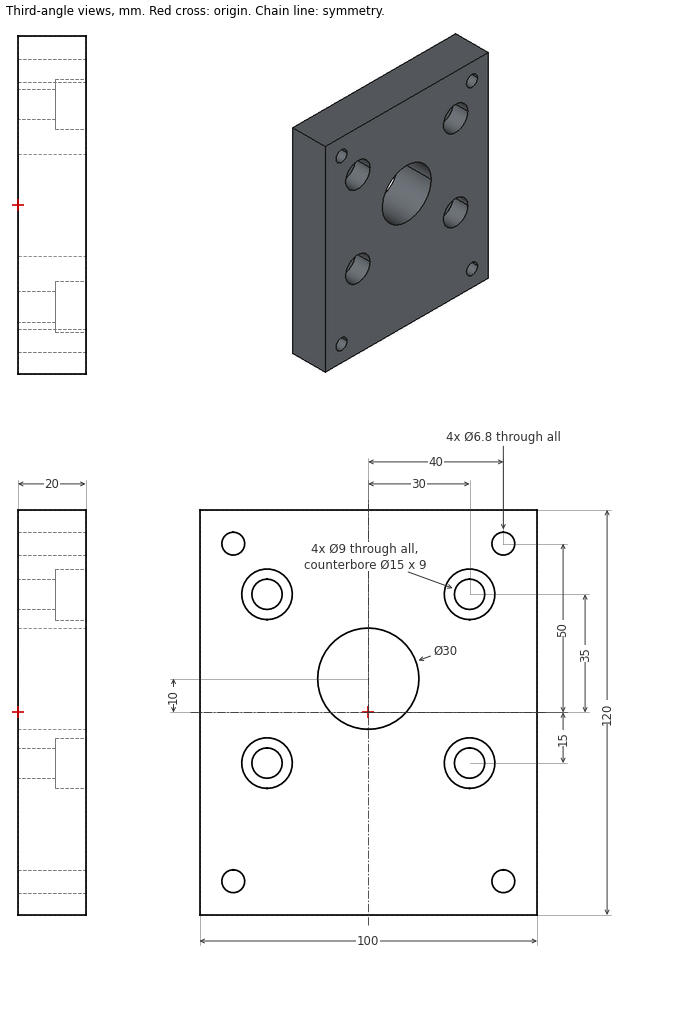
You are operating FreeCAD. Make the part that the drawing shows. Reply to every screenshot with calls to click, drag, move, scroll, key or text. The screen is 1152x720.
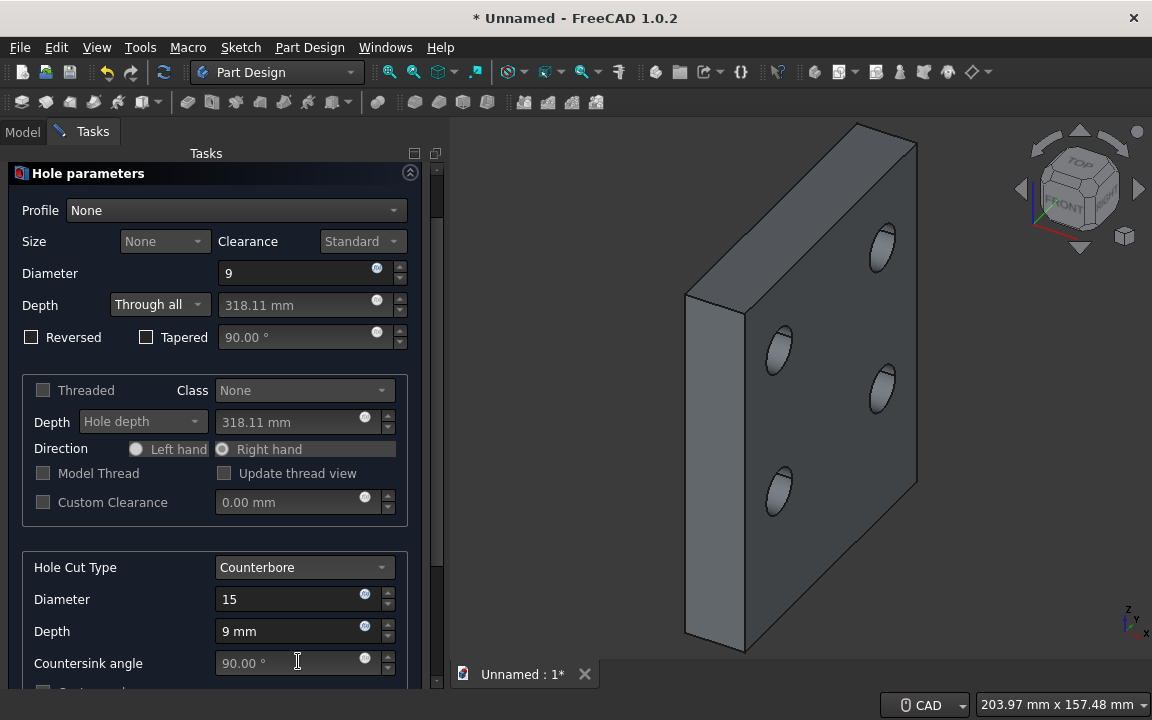
scroll(437, 426, up, 2)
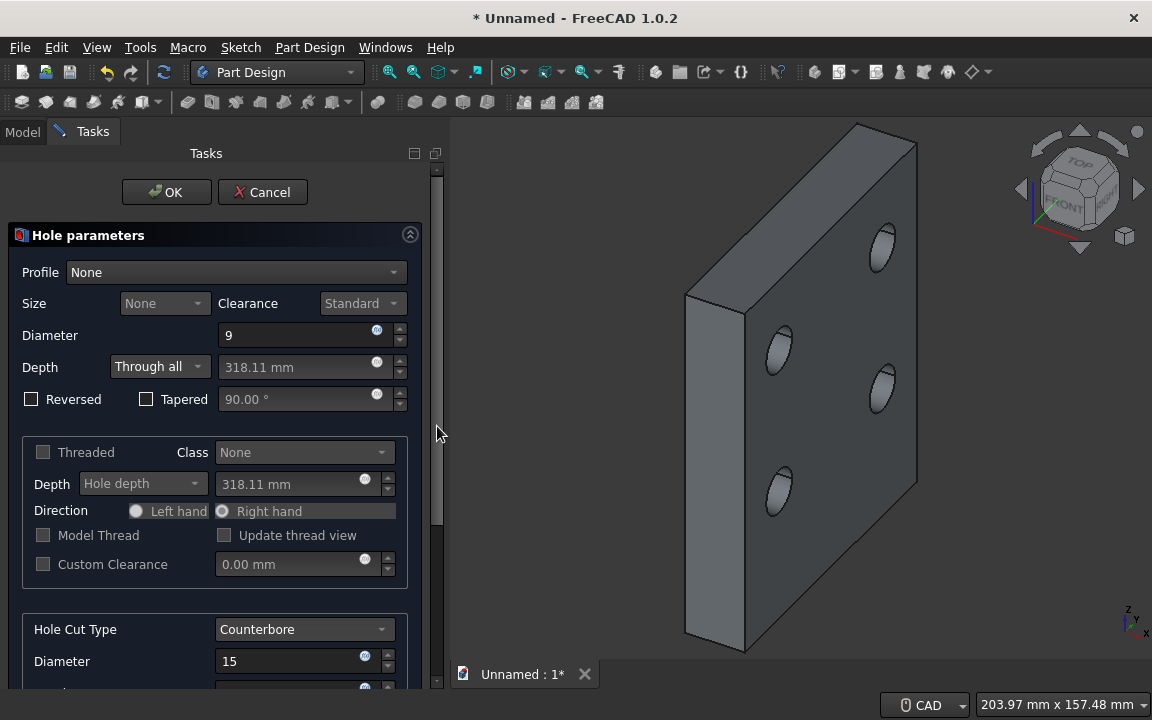
click(167, 192)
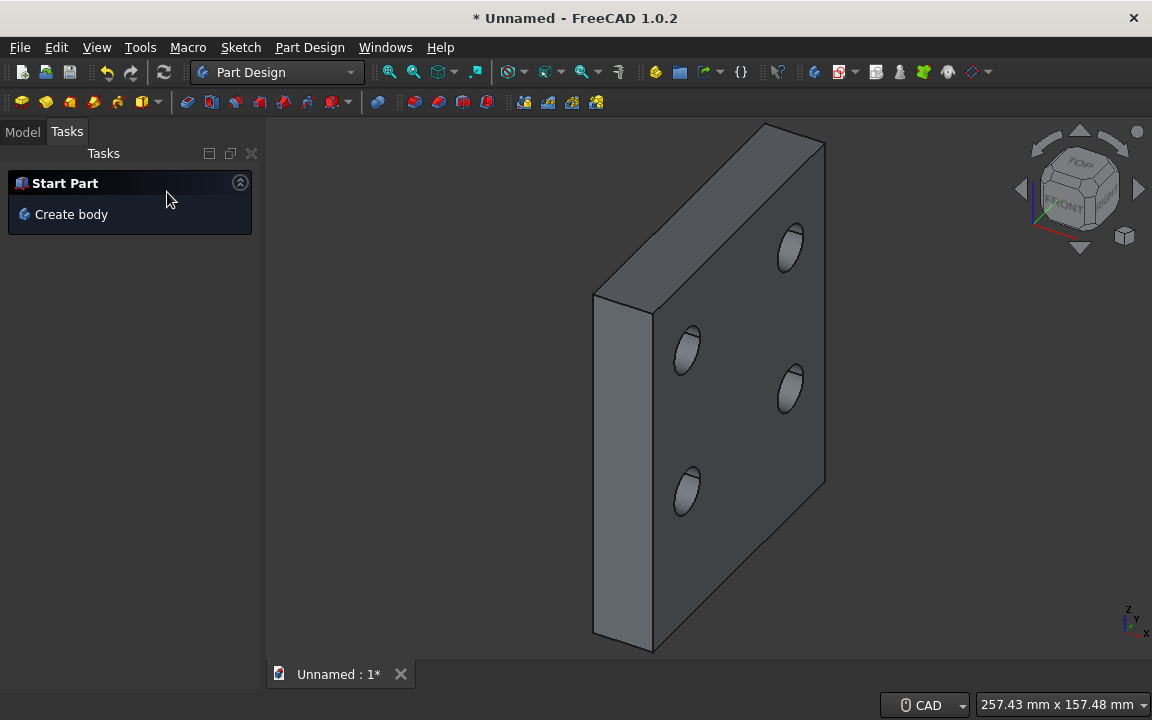
click(739, 349)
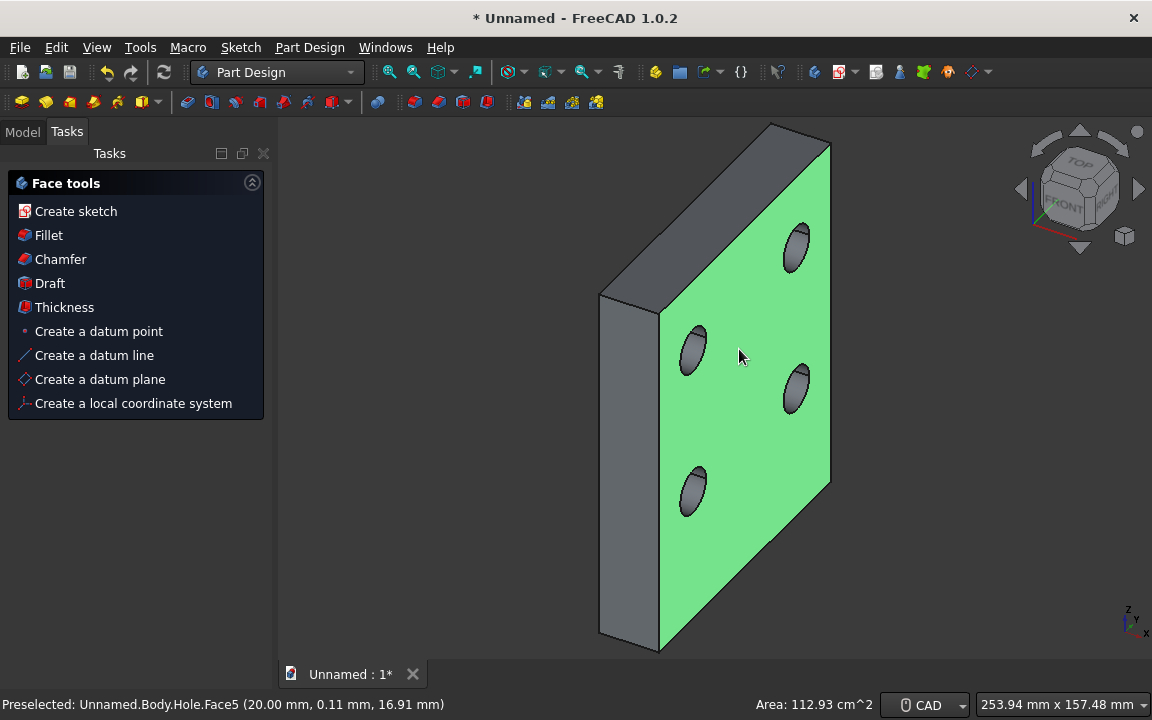
click(840, 72)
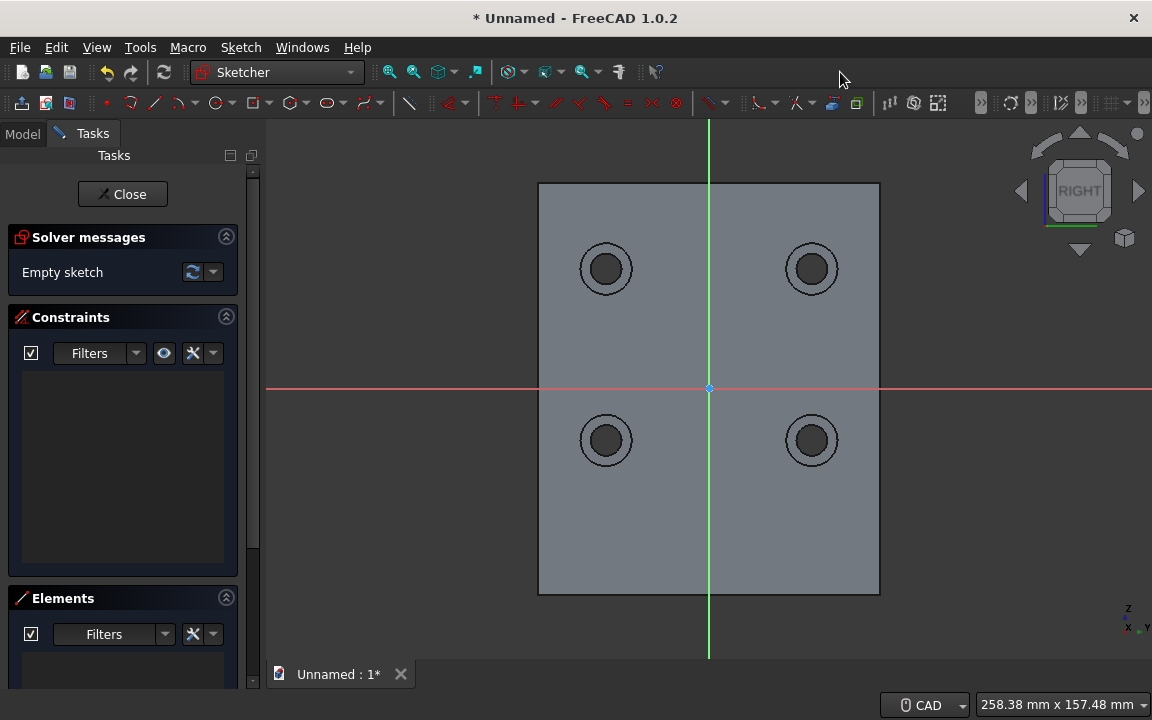
scroll(739, 340, up, 6)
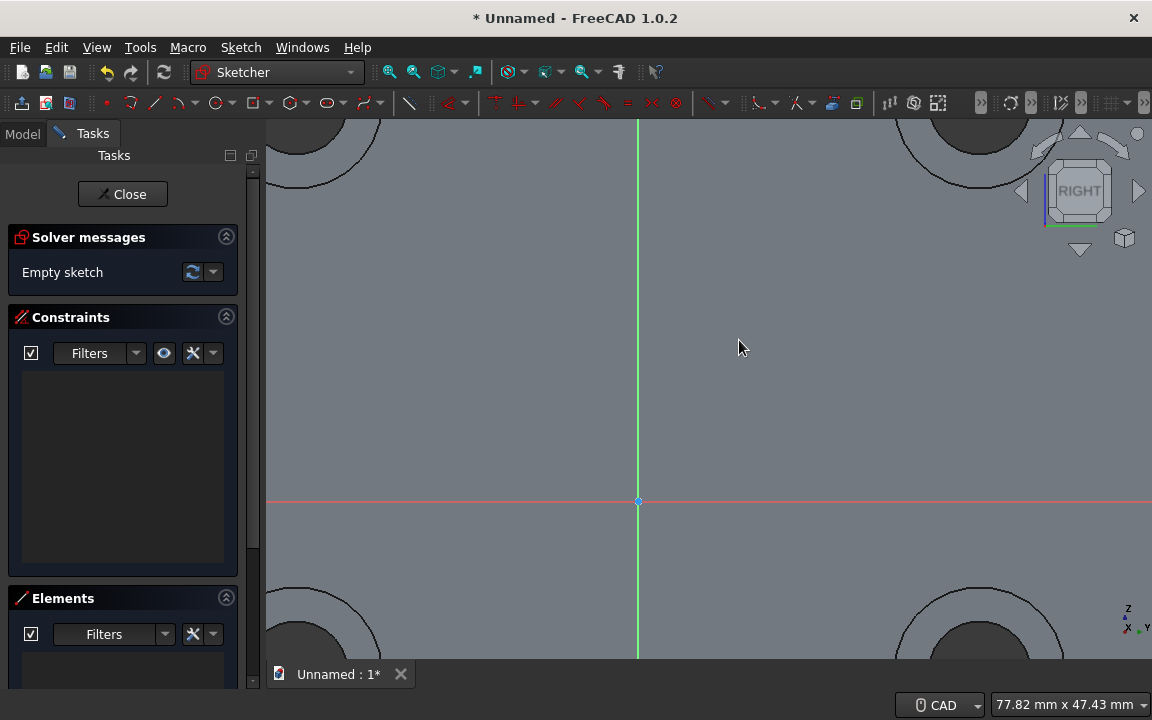
click(216, 104)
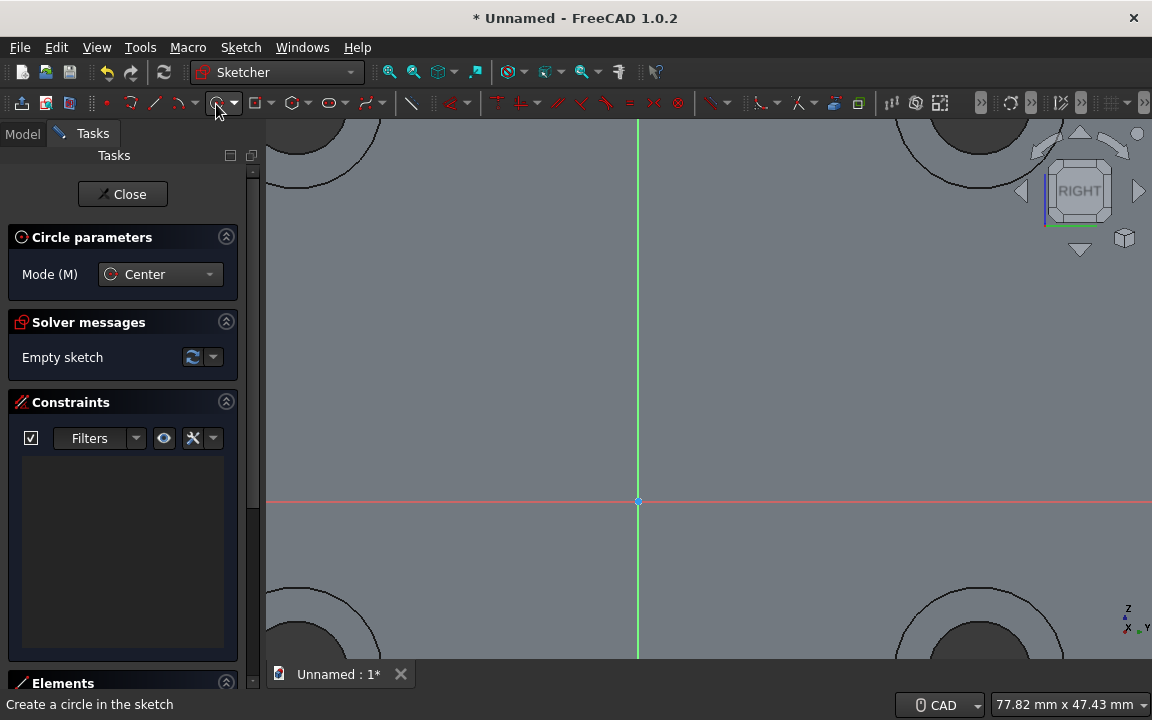
click(638, 388)
click(759, 267)
key(Escape)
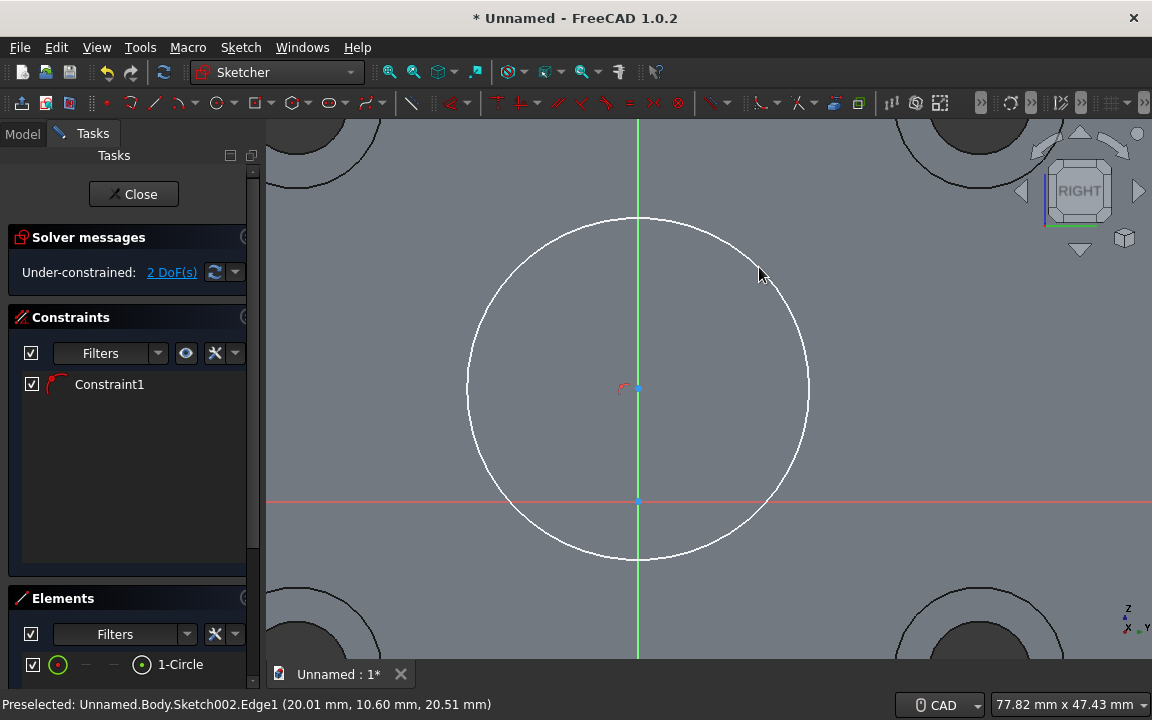
click(450, 104)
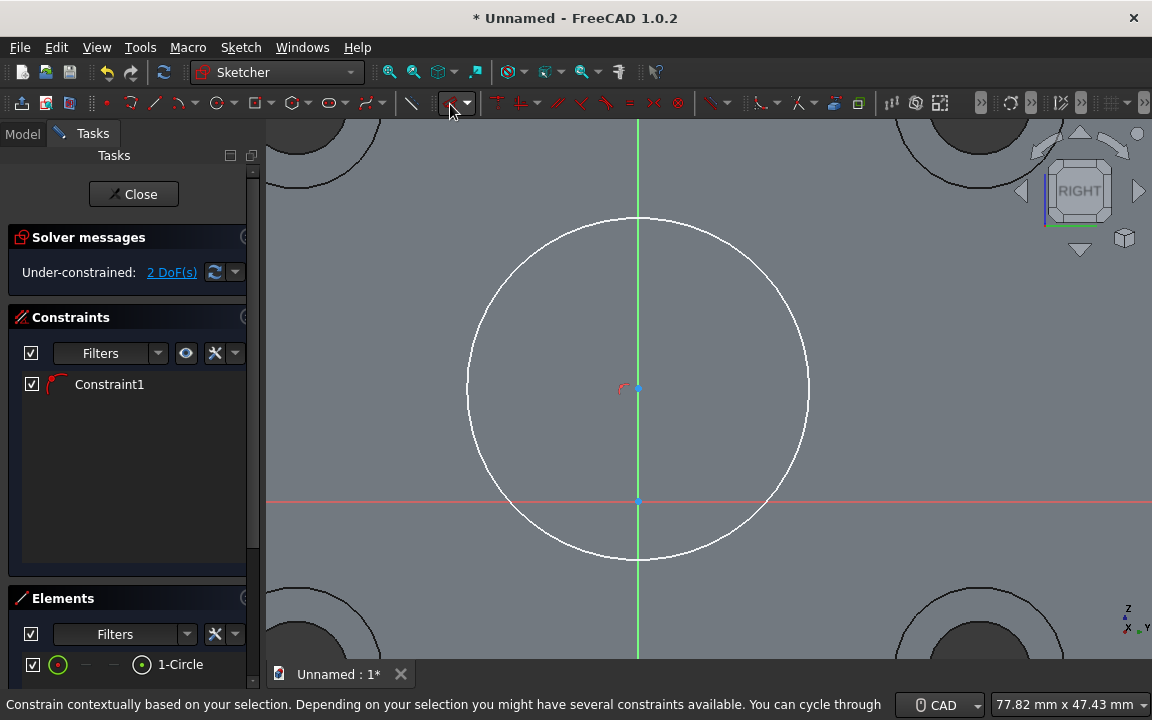
click(759, 268)
click(782, 245)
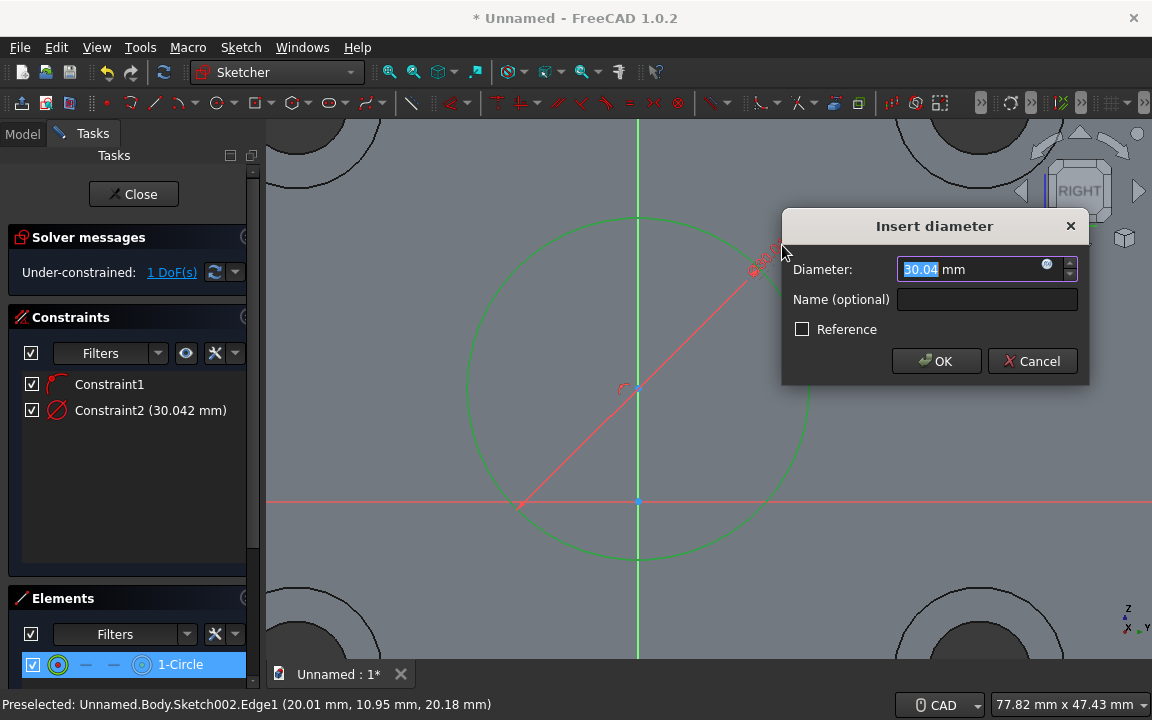
text(30)
key(Return)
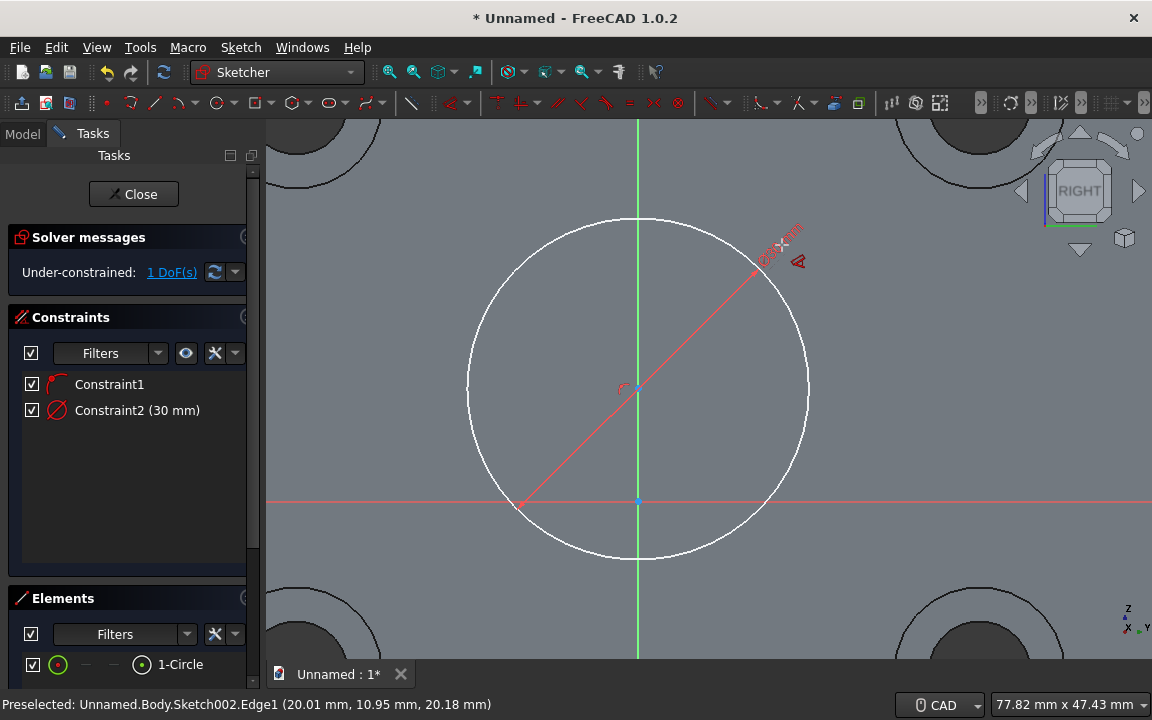
click(638, 389)
click(672, 445)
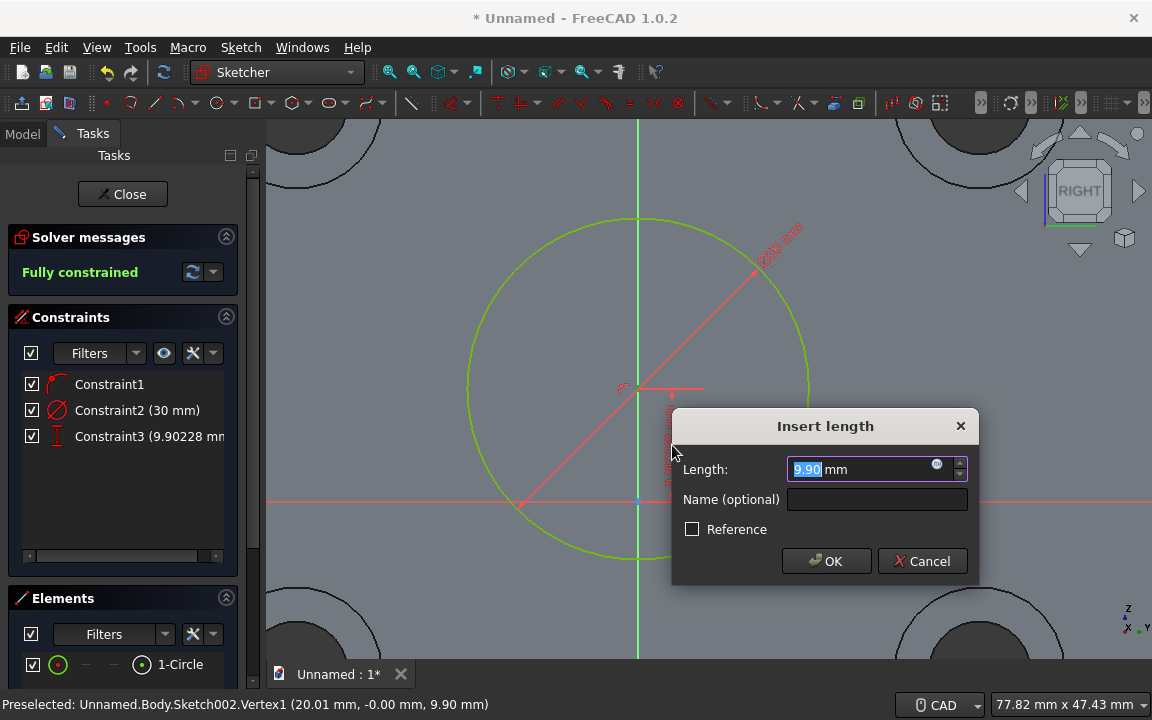
text(10)
key(Return)
key(Escape)